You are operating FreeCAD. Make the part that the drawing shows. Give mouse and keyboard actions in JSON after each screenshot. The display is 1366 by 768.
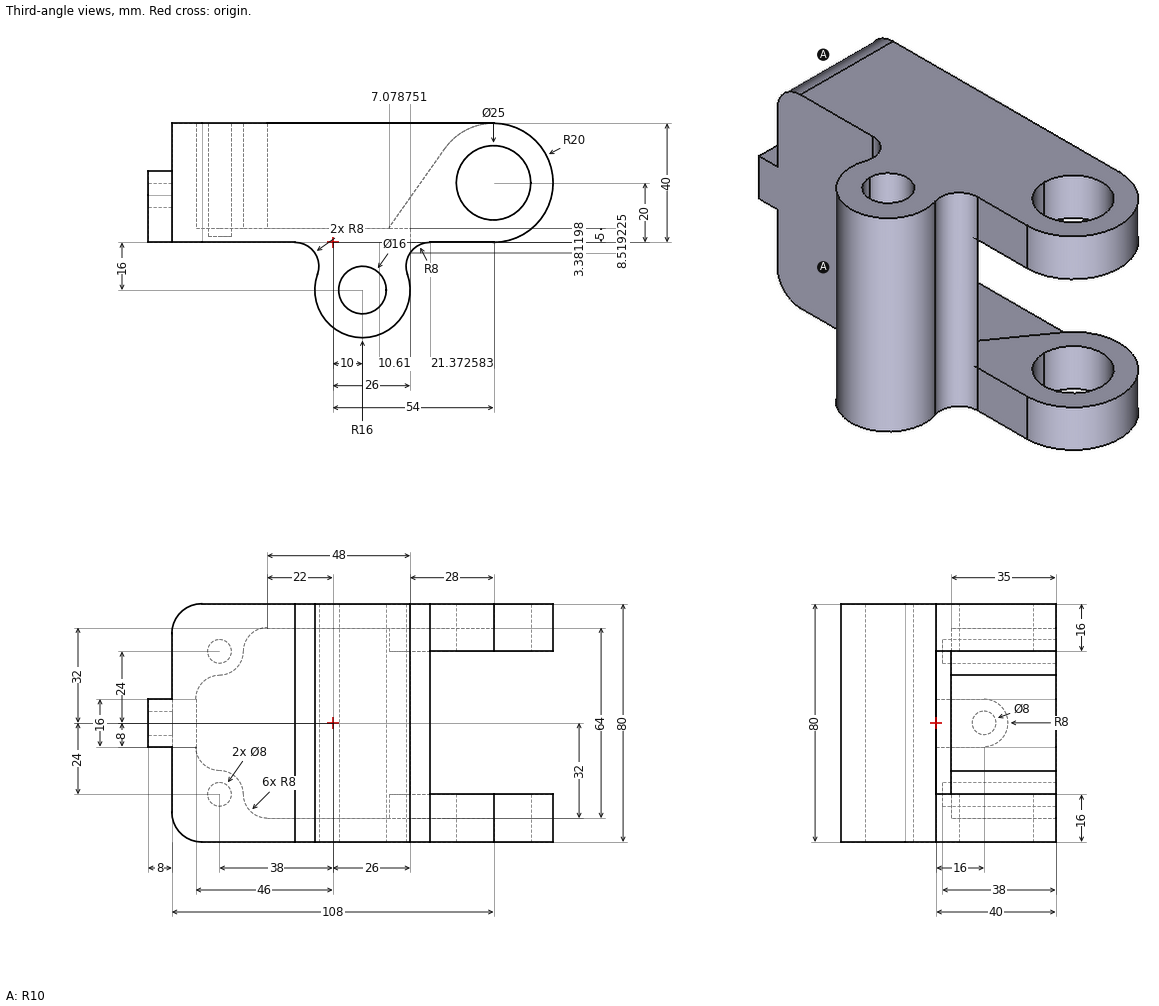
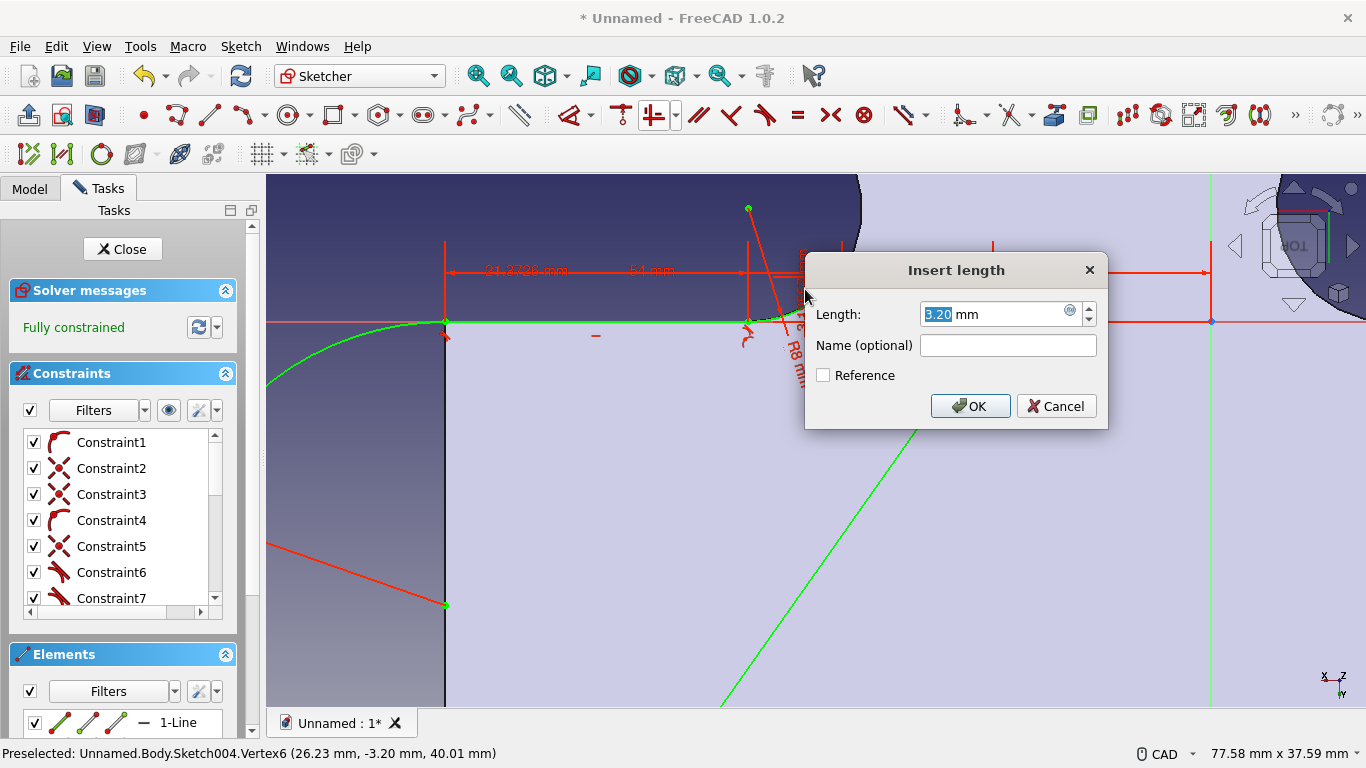
{"action": "type", "text": "3.381198"}
{"action": "key", "text": "Return"}
{"action": "key", "text": "Escape"}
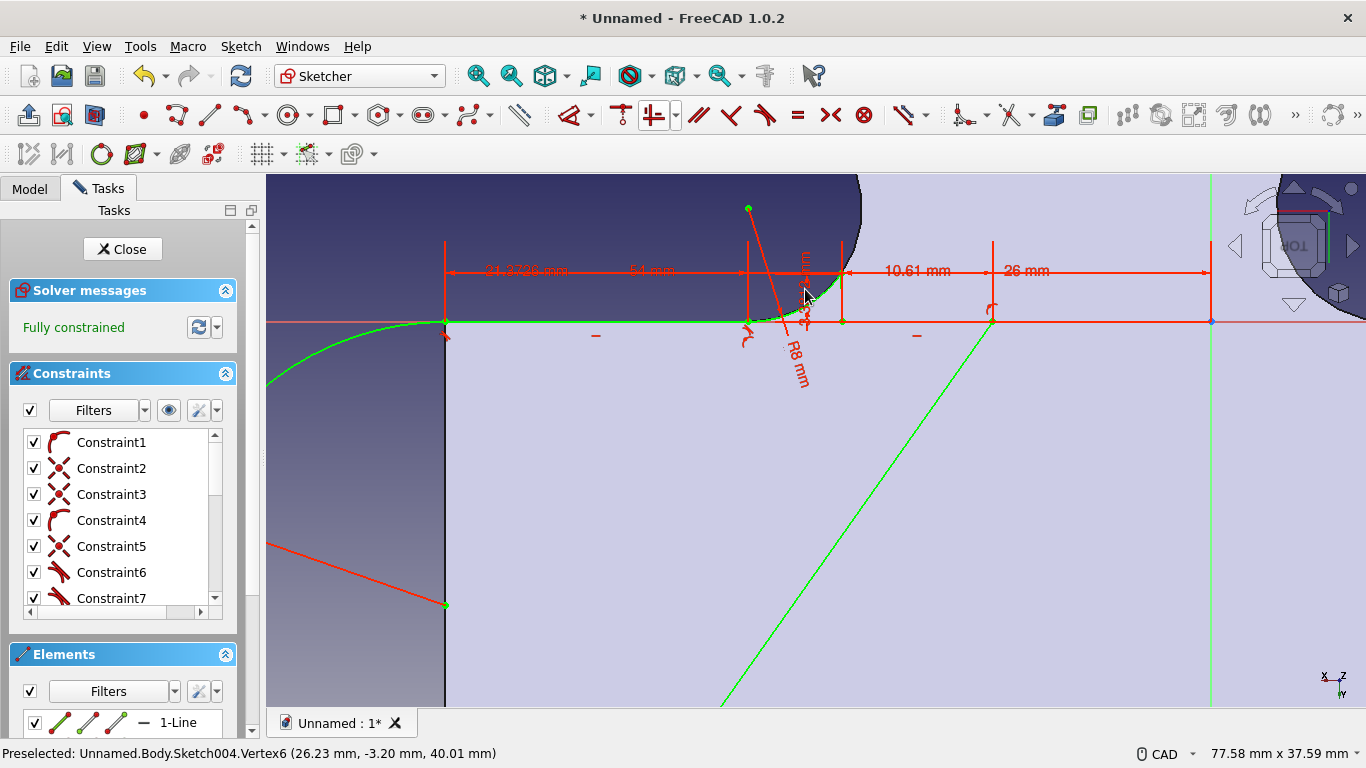
{"action": "left_click", "coordinate": [123, 249]}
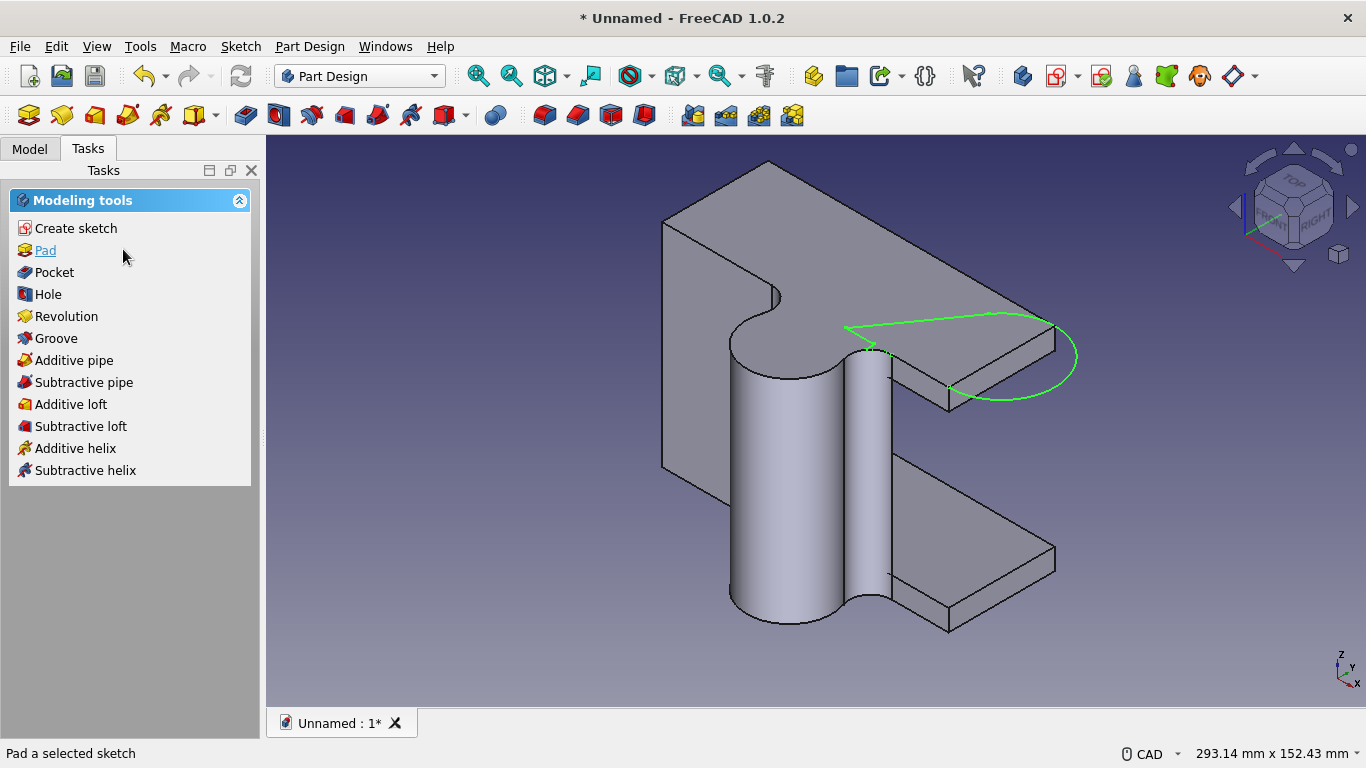
{"action": "left_click", "coordinate": [29, 116]}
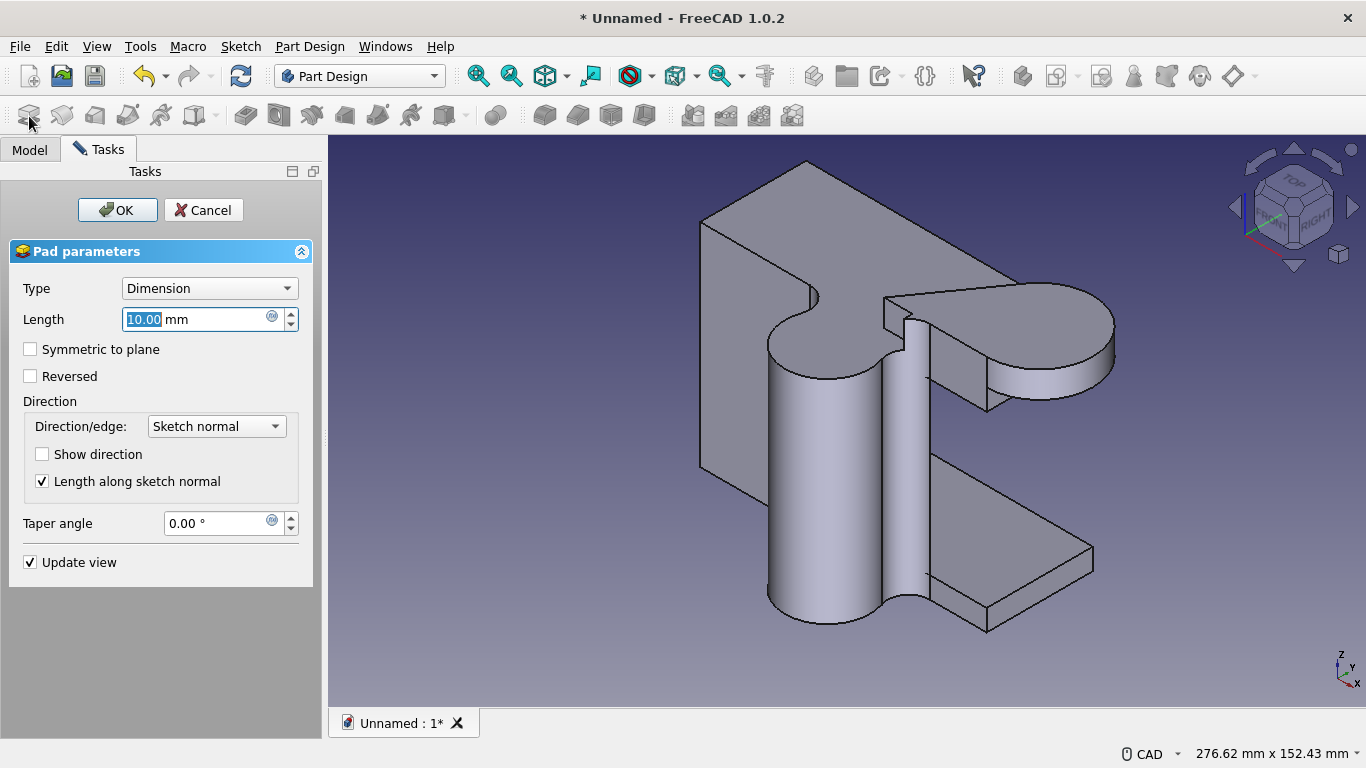
{"action": "type", "text": "16"}
{"action": "key", "text": "Tab"}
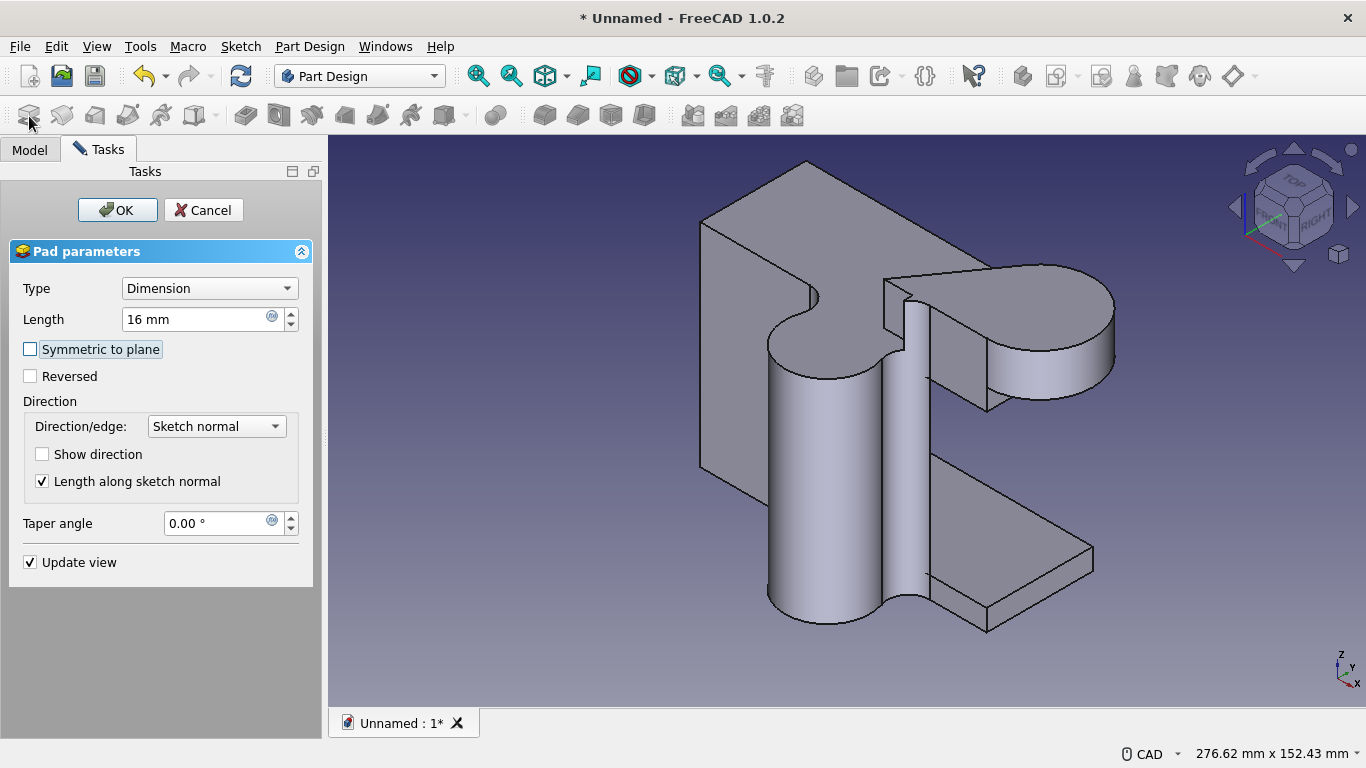
{"action": "left_click", "coordinate": [31, 376]}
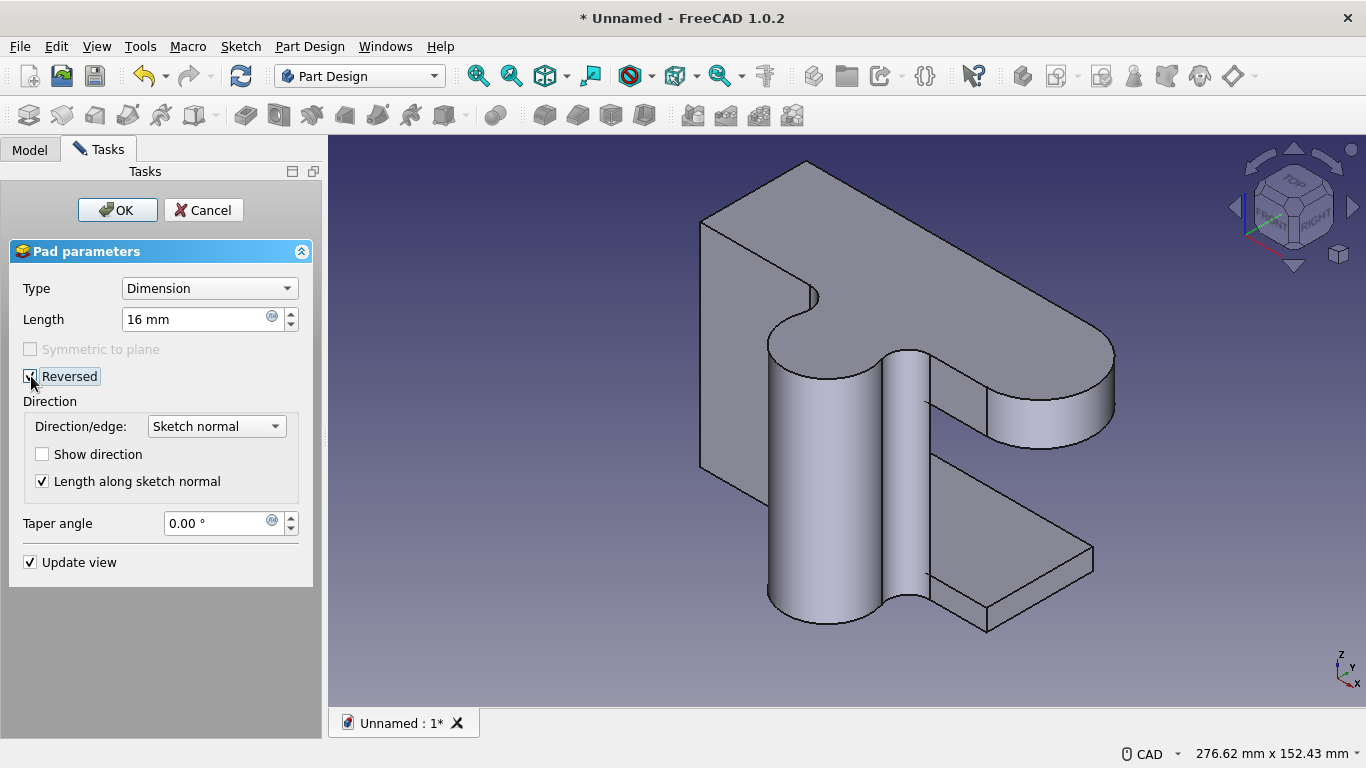
{"action": "left_click", "coordinate": [118, 210]}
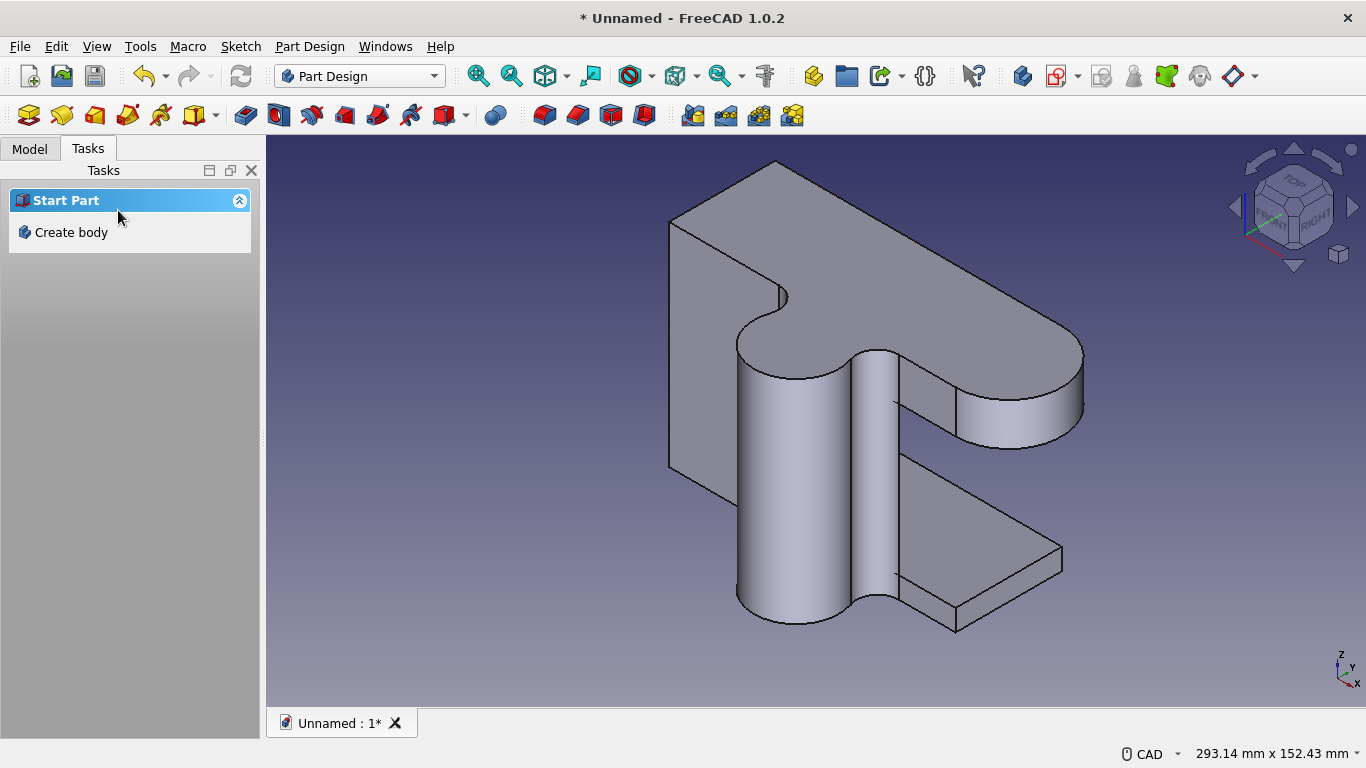
{"action": "left_click", "coordinate": [479, 76]}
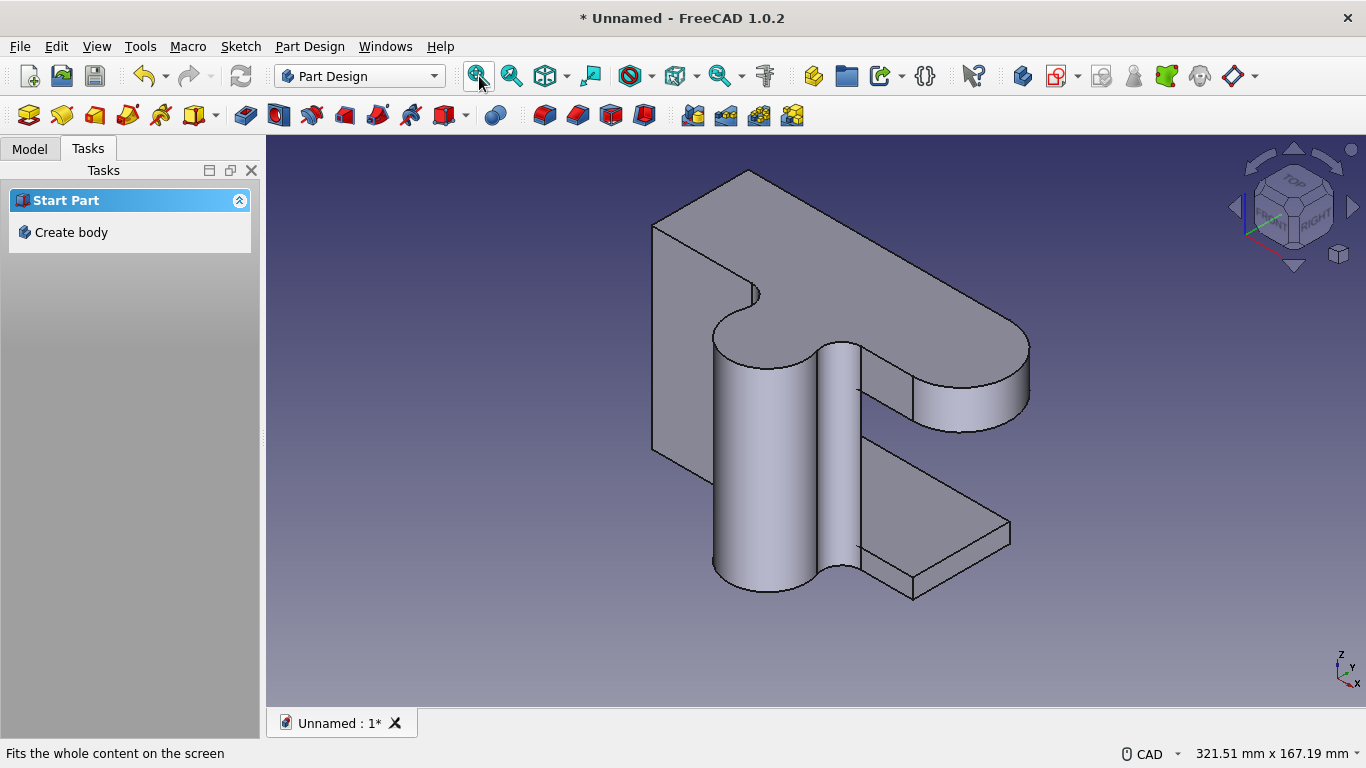
{"action": "left_click", "coordinate": [30, 148]}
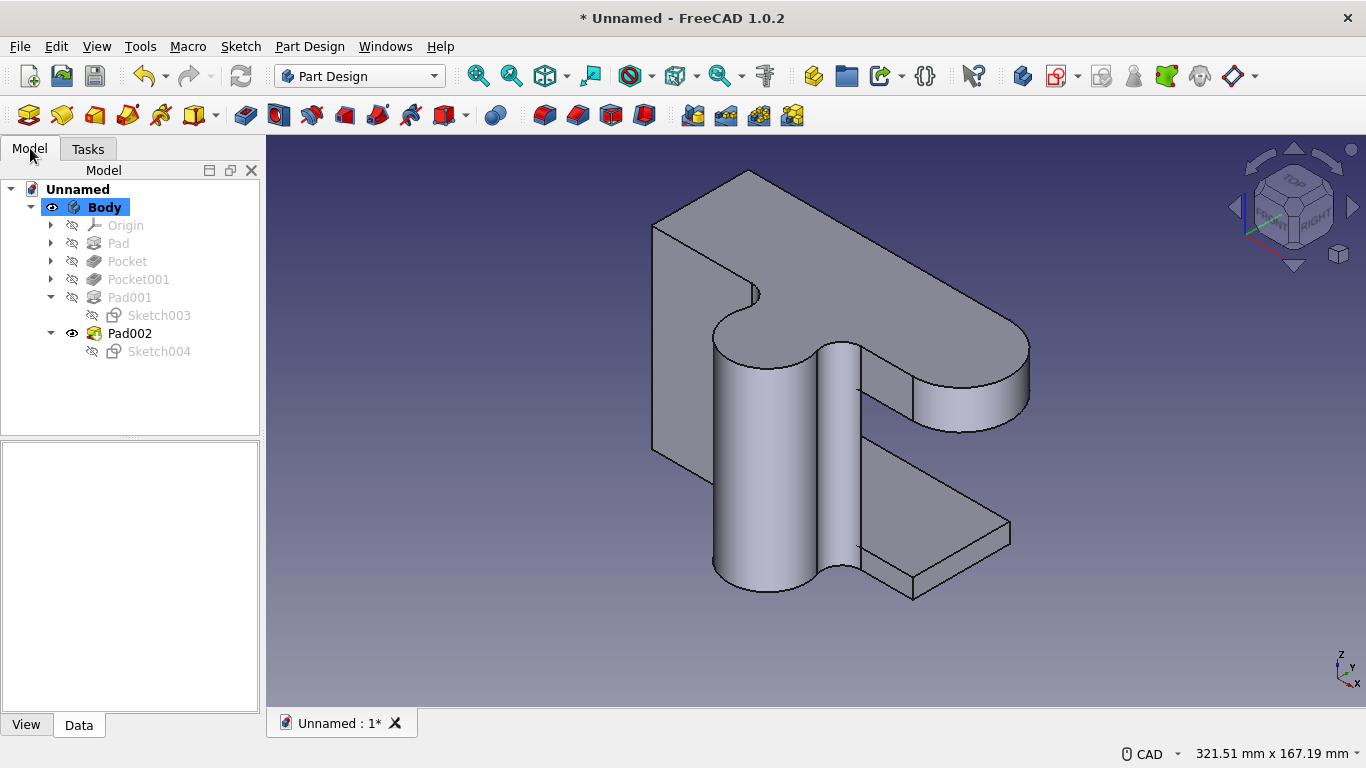
{"action": "left_click", "coordinate": [51, 225]}